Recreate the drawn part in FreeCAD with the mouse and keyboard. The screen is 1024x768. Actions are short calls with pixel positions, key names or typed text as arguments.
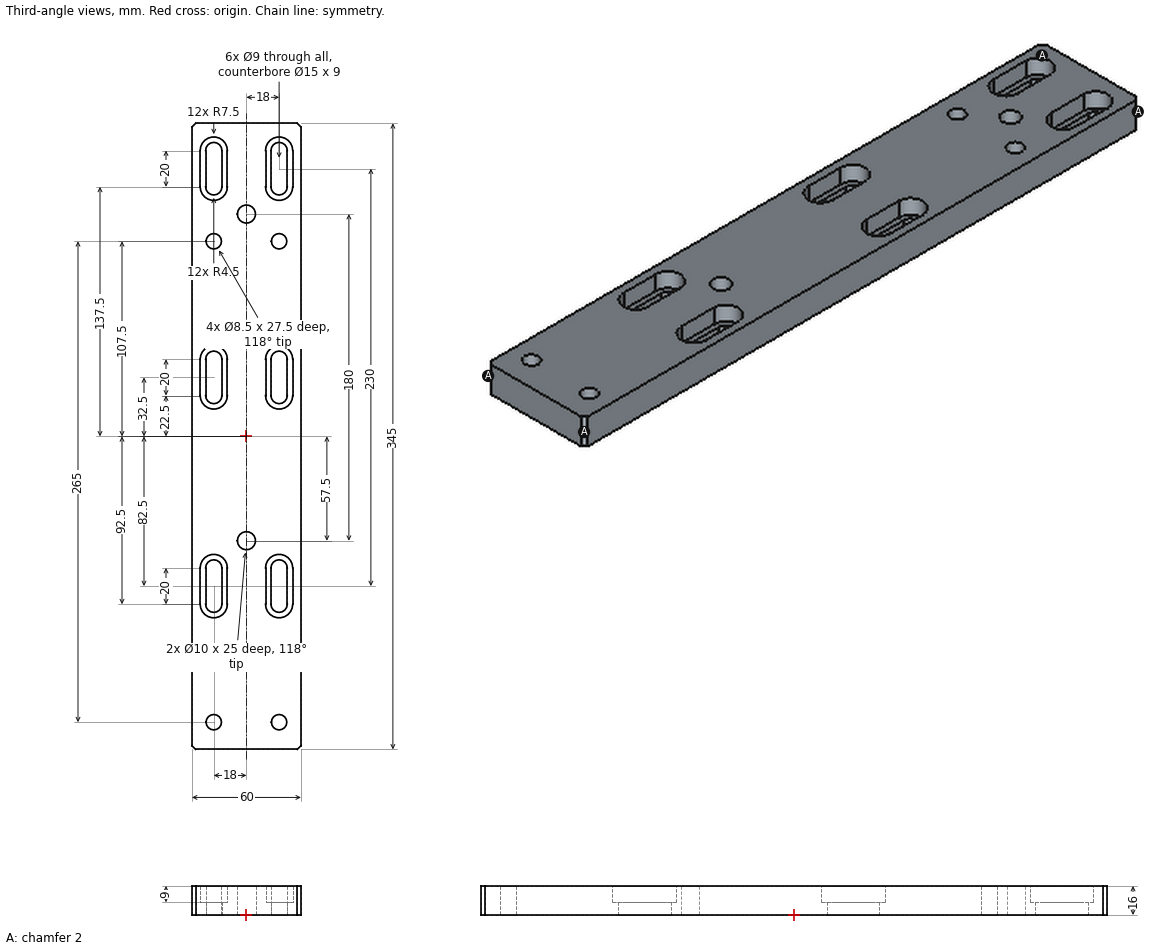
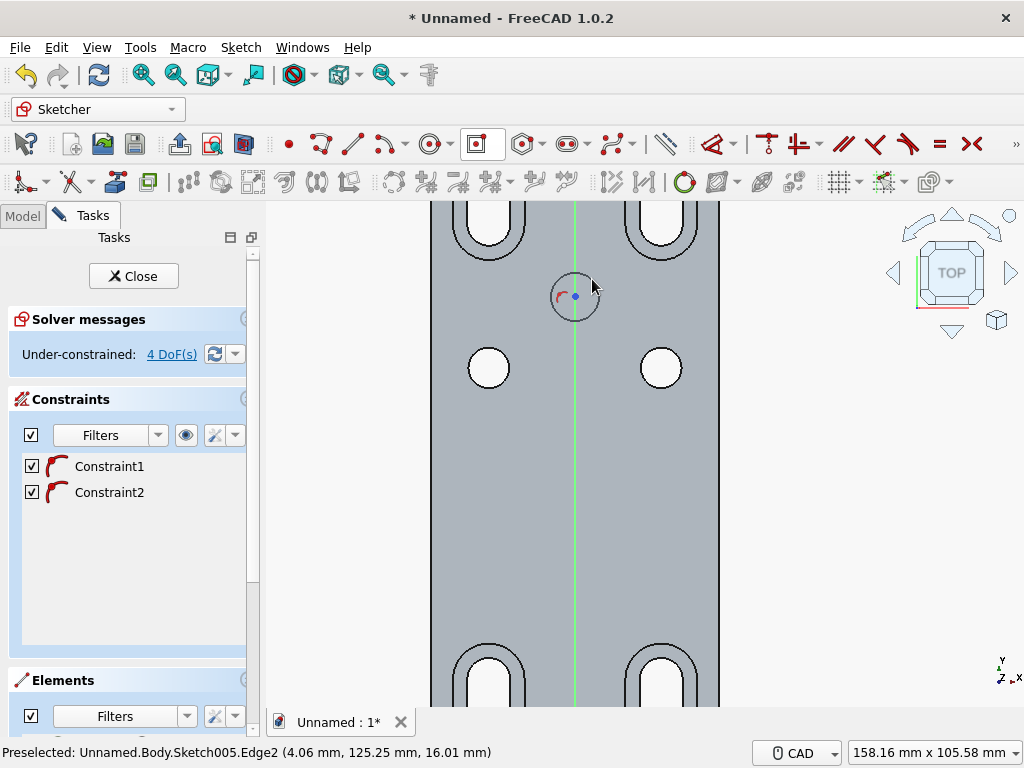
scroll(577, 295, down, 5)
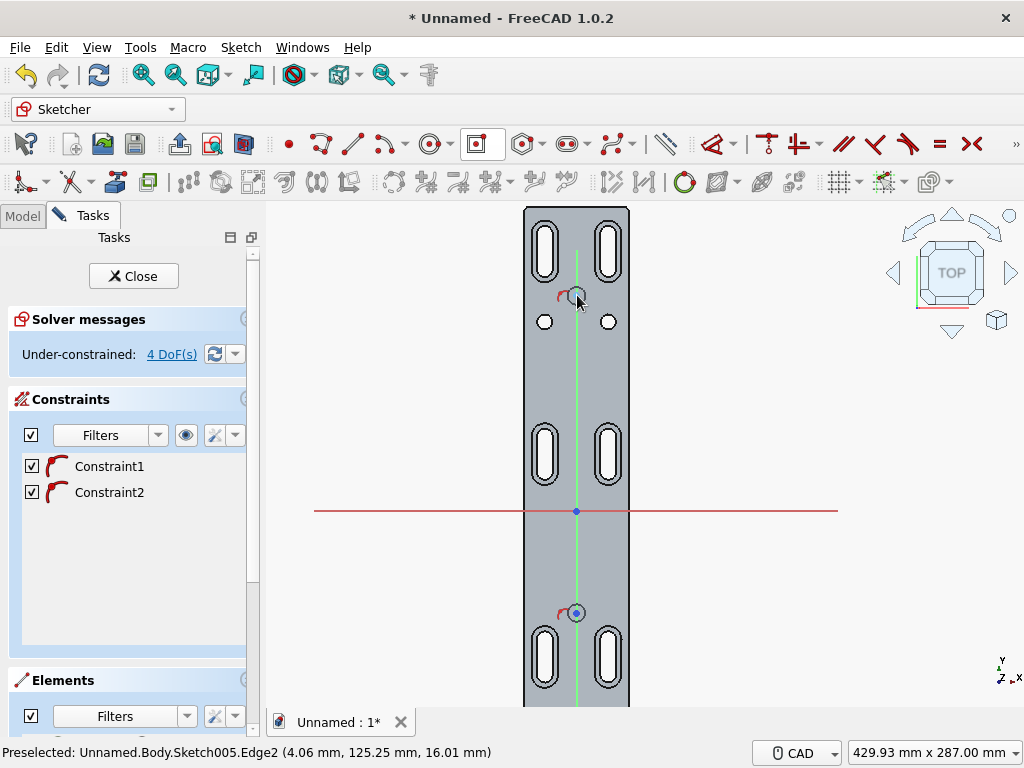
scroll(583, 607, up, 5)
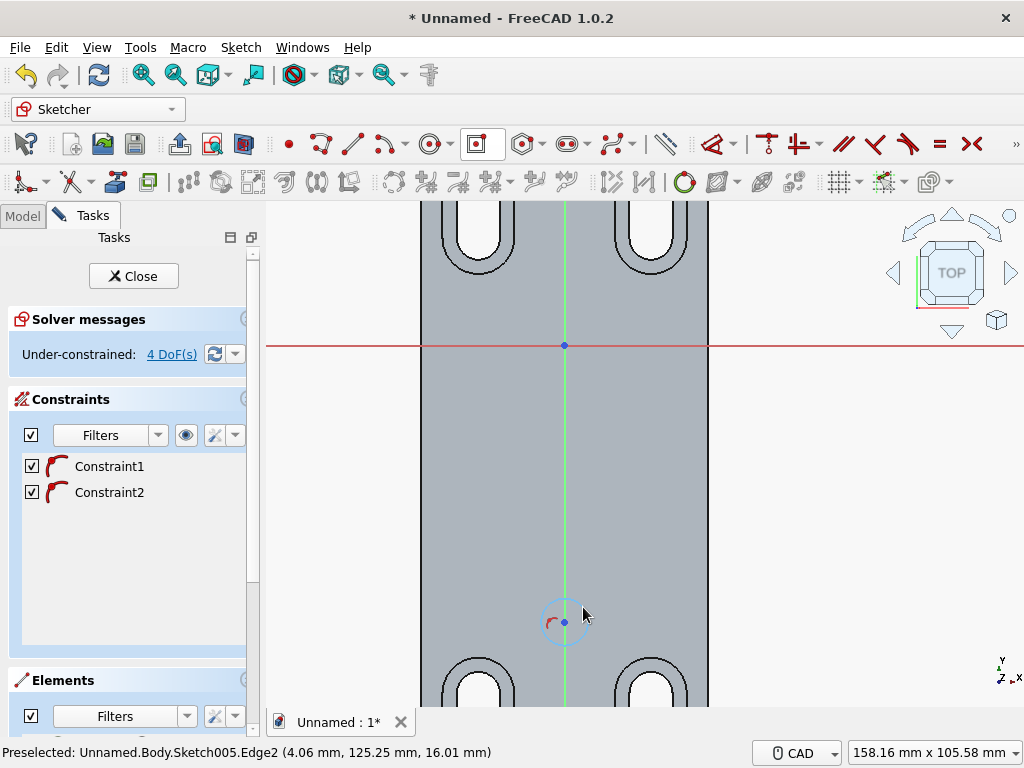
click(581, 605)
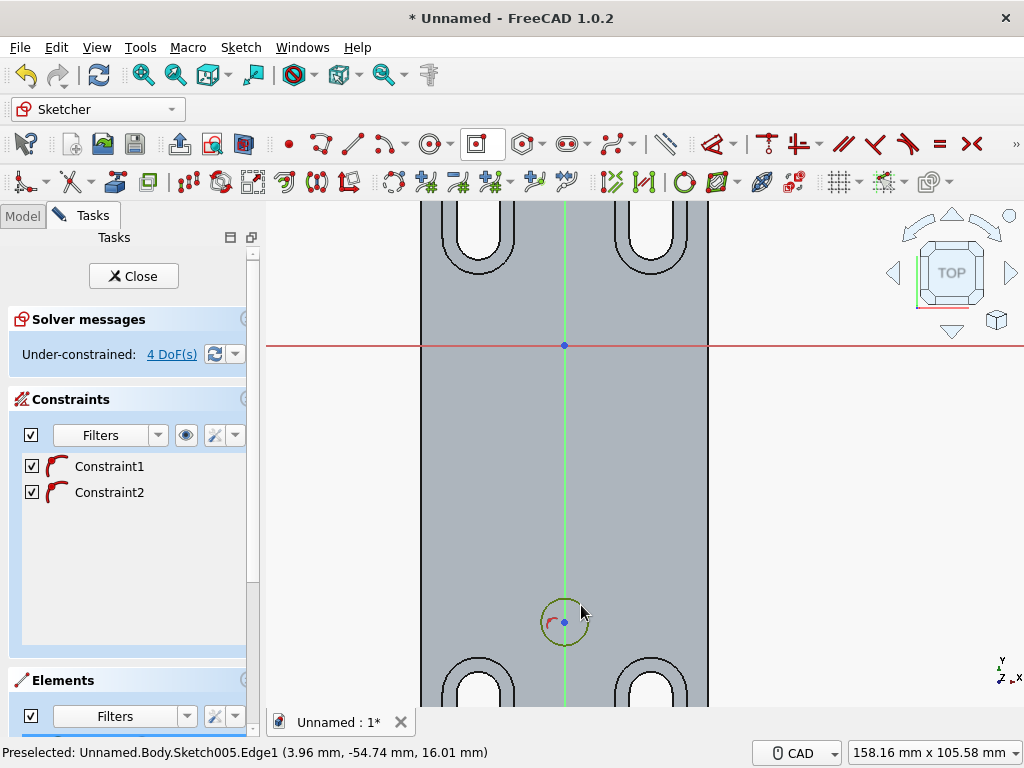
scroll(583, 608, down, 5)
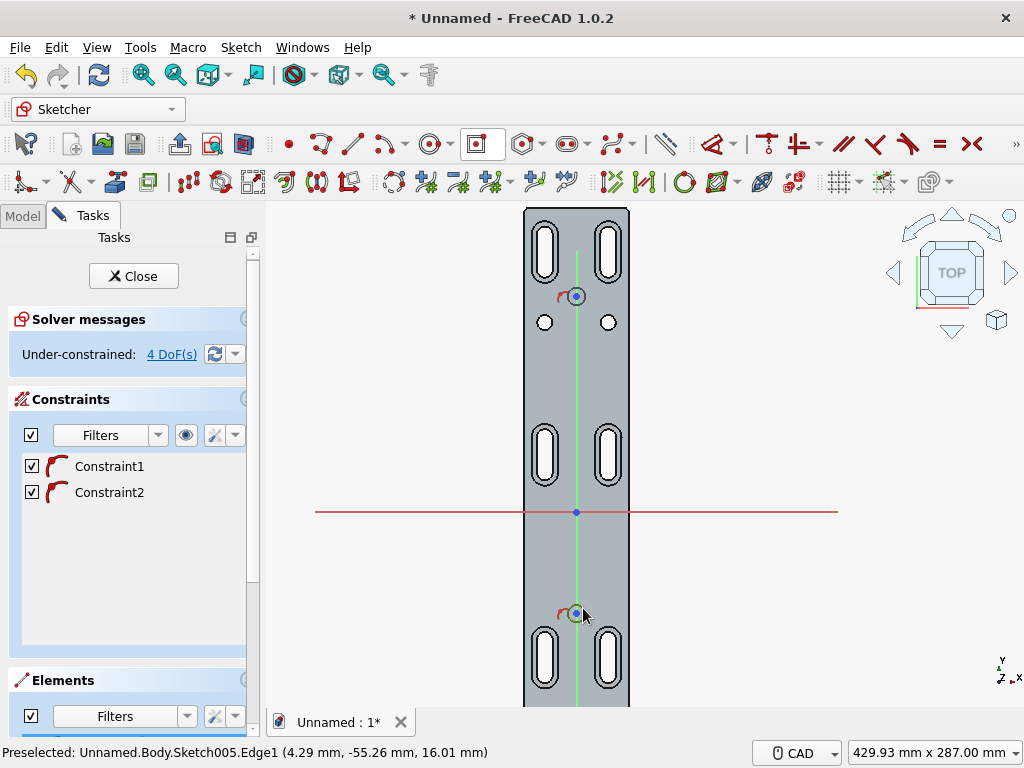
scroll(583, 290, up, 4)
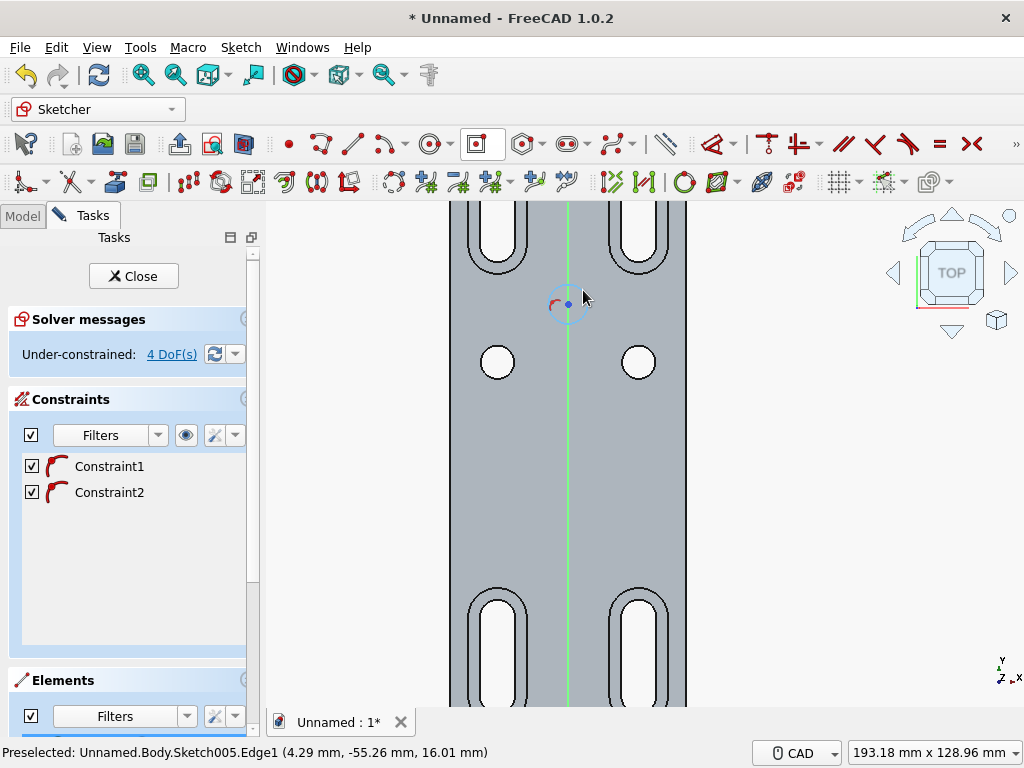
click(582, 290)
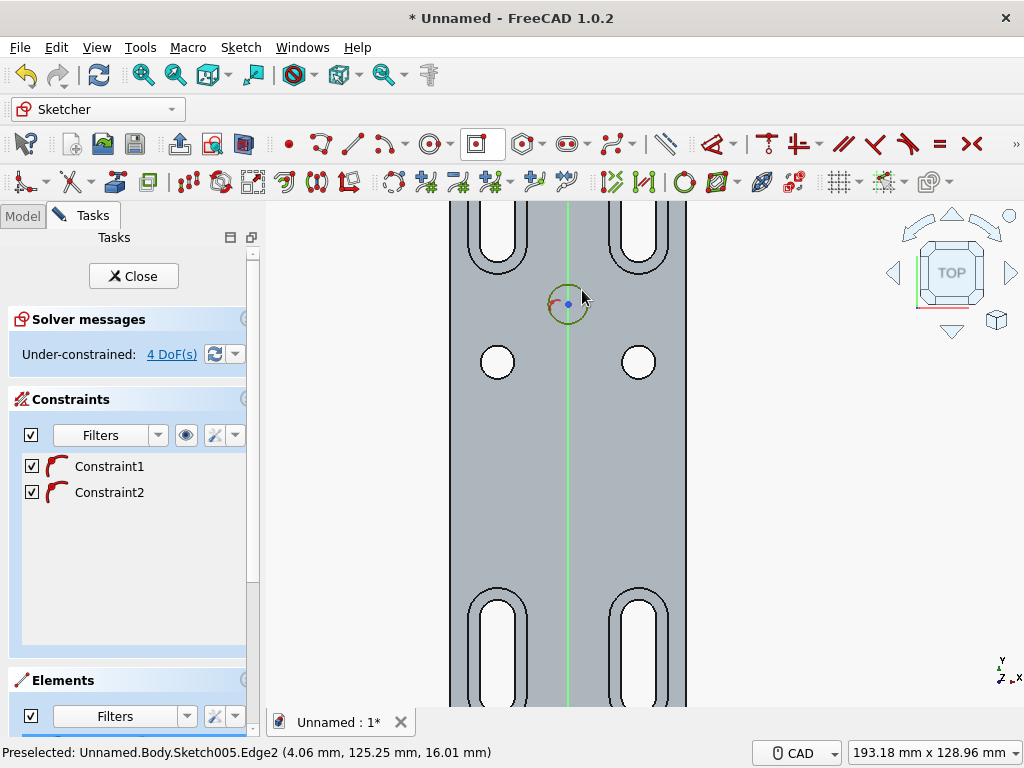
click(940, 144)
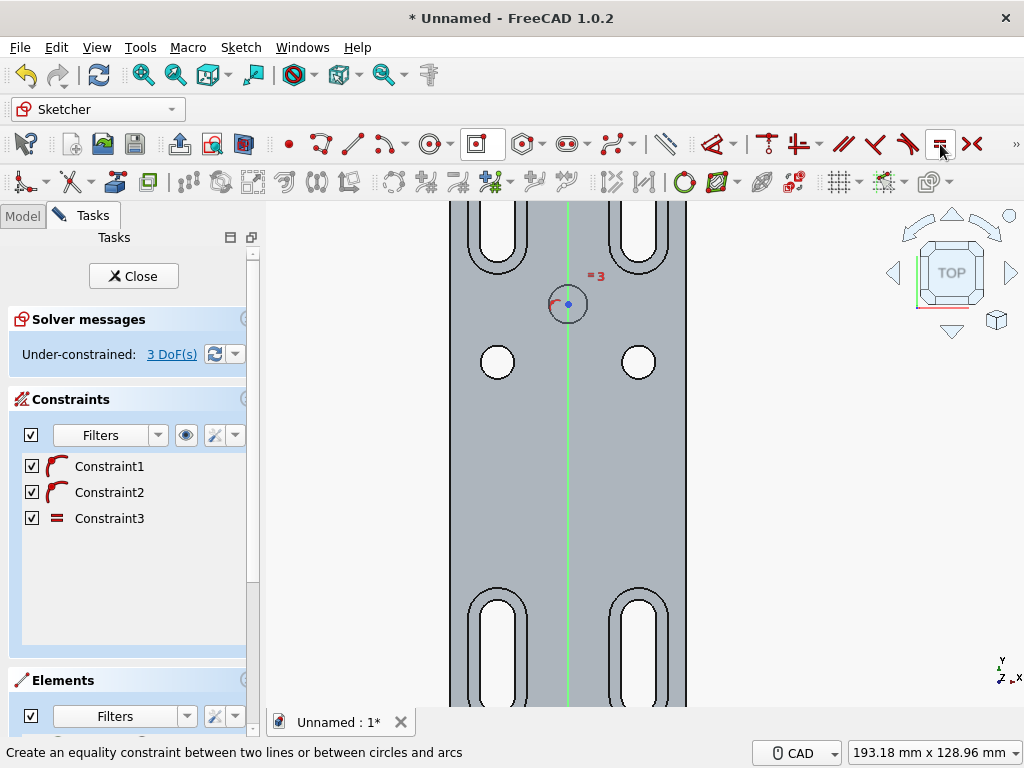
key(d)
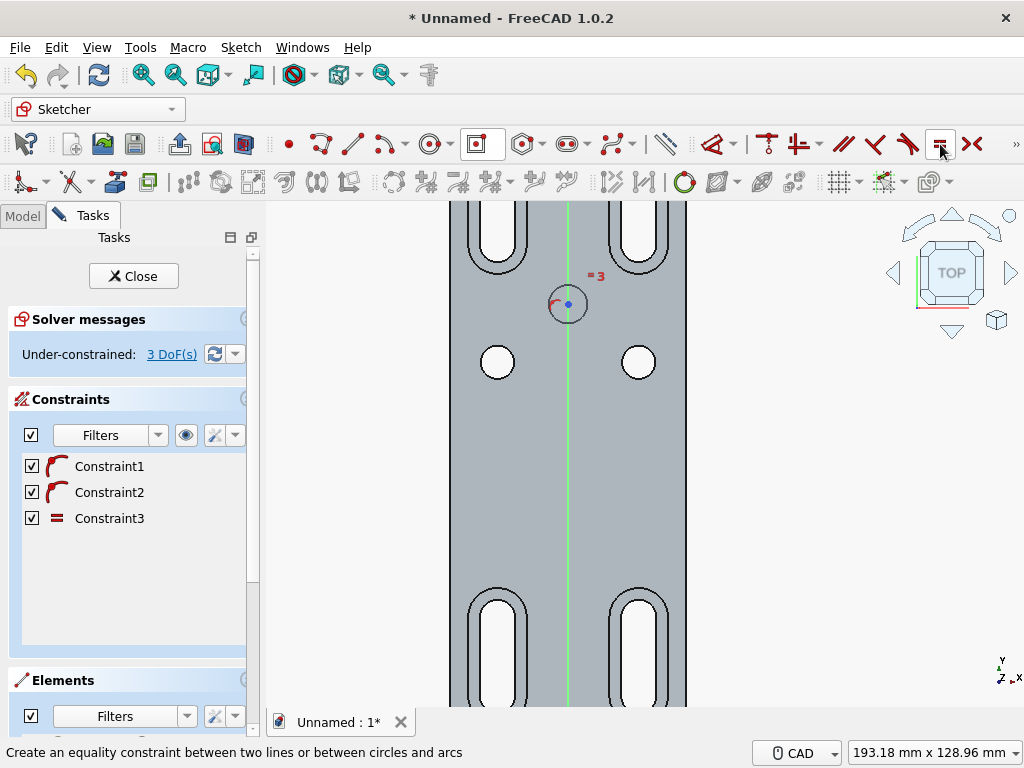
scroll(583, 289, down, 4)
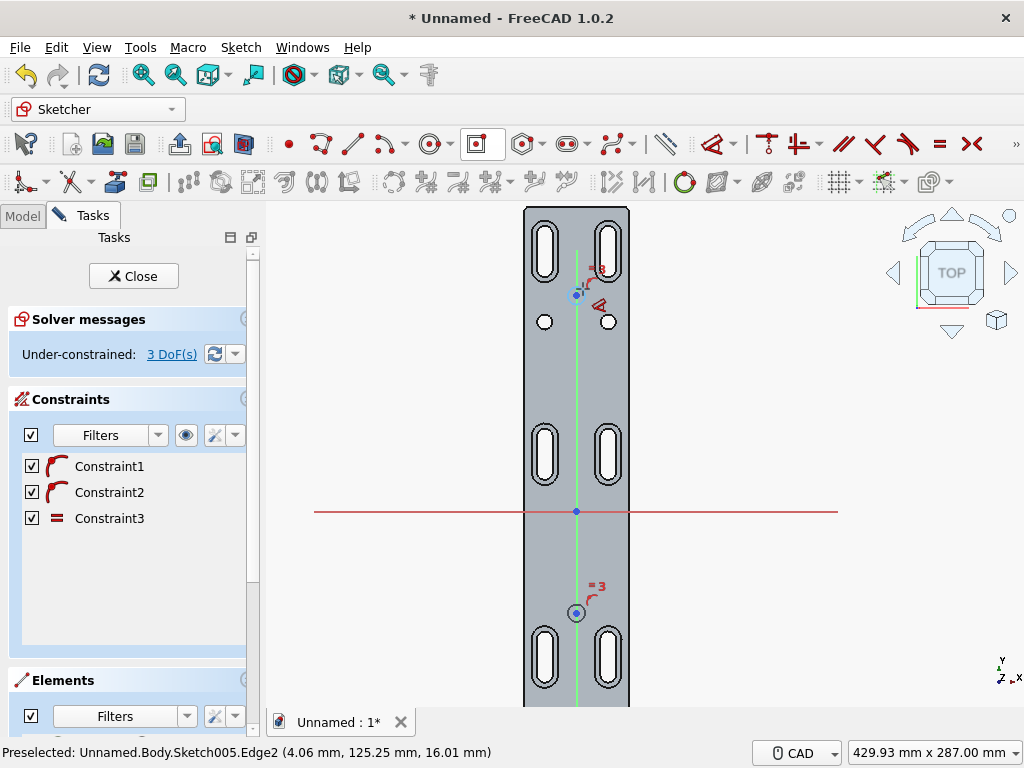
scroll(583, 607, up, 5)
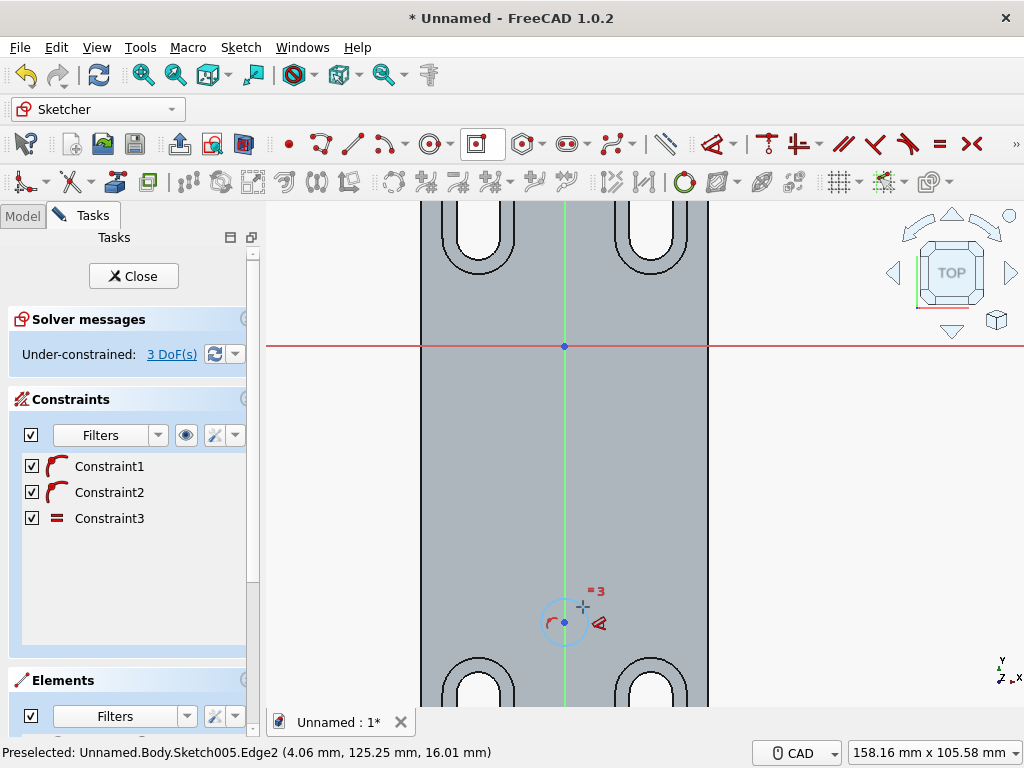
click(581, 606)
click(604, 583)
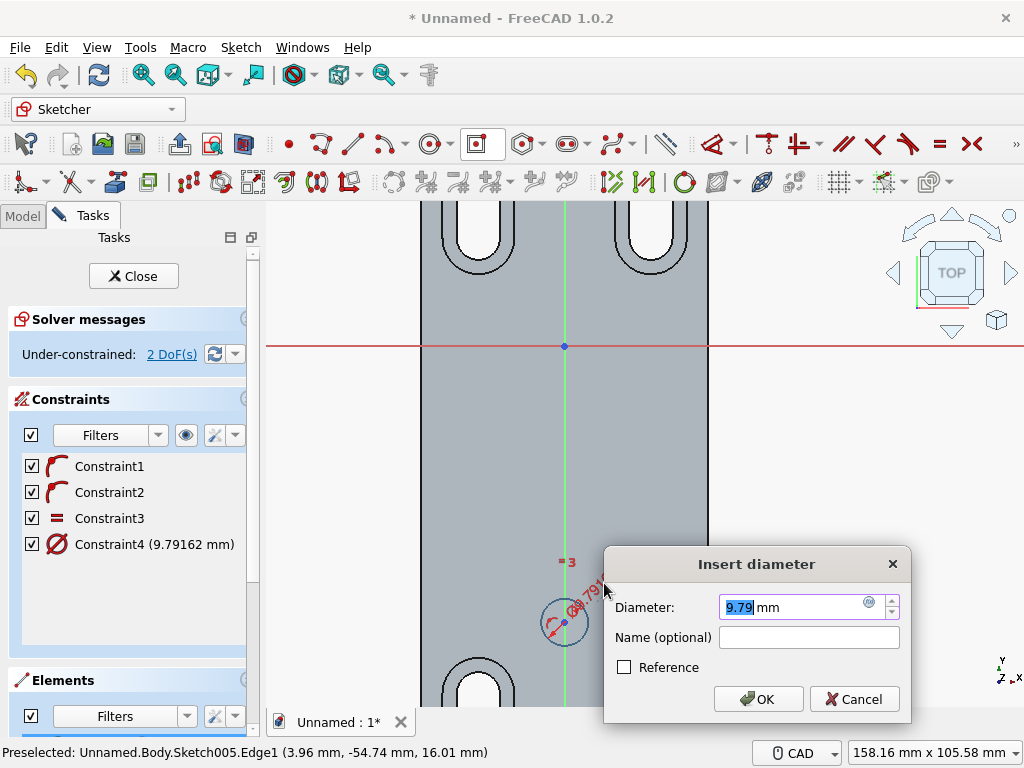
text(10)
key(Return)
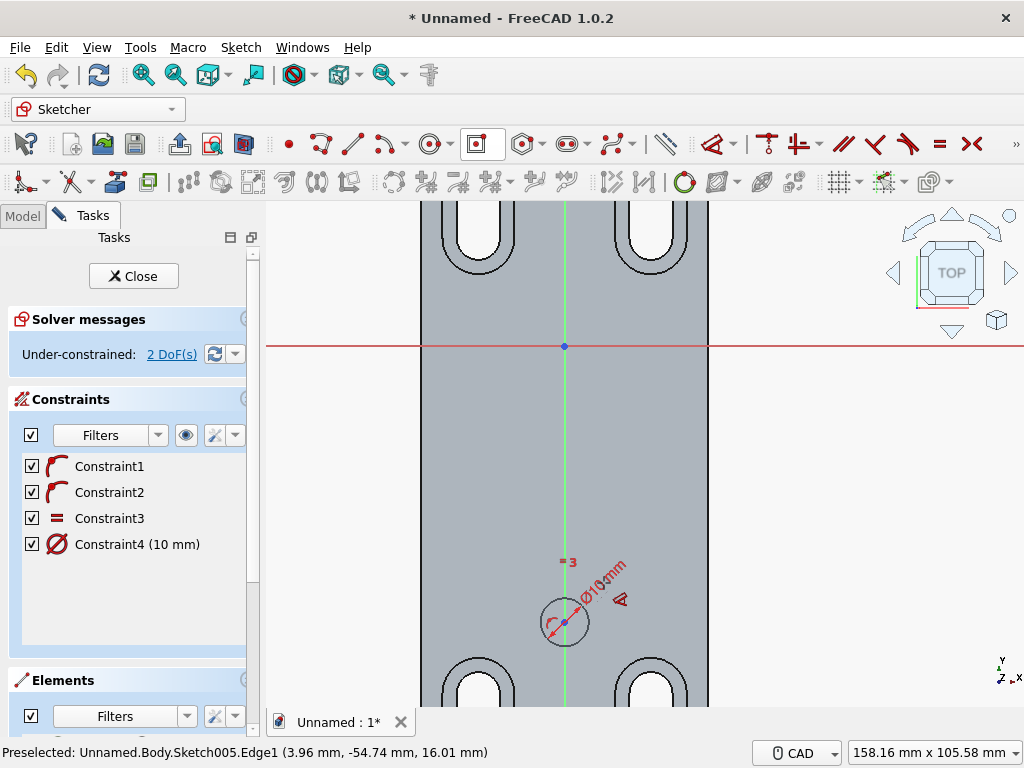
click(565, 622)
click(599, 484)